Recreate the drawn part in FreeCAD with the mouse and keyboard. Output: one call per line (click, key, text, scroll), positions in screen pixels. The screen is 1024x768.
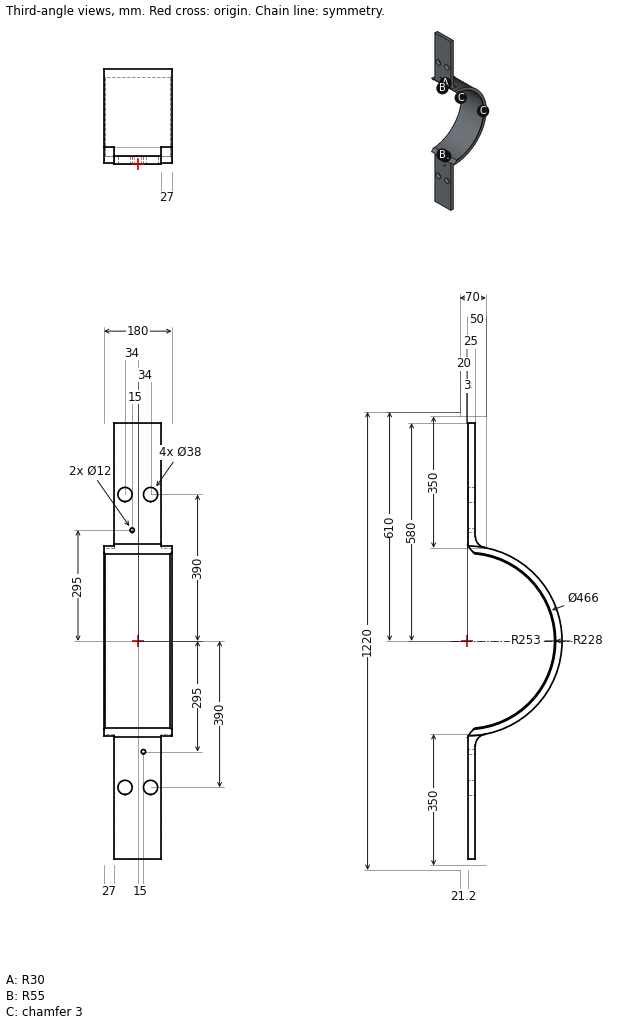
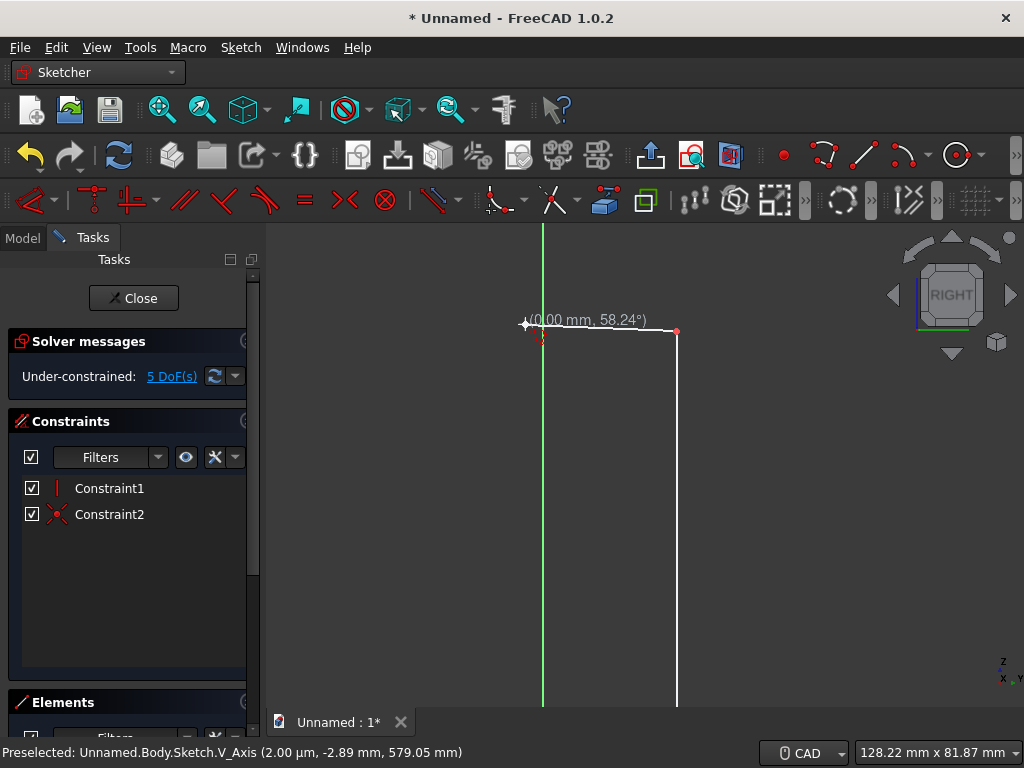
scroll(540, 293, down, 15)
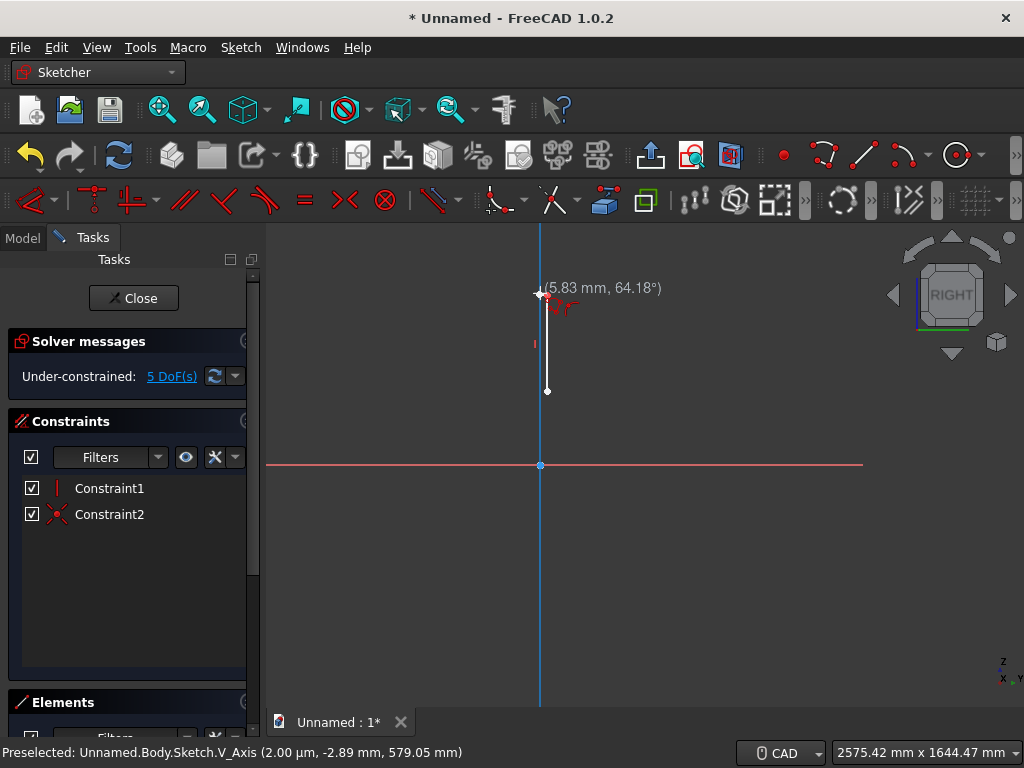
scroll(540, 398, up, 15)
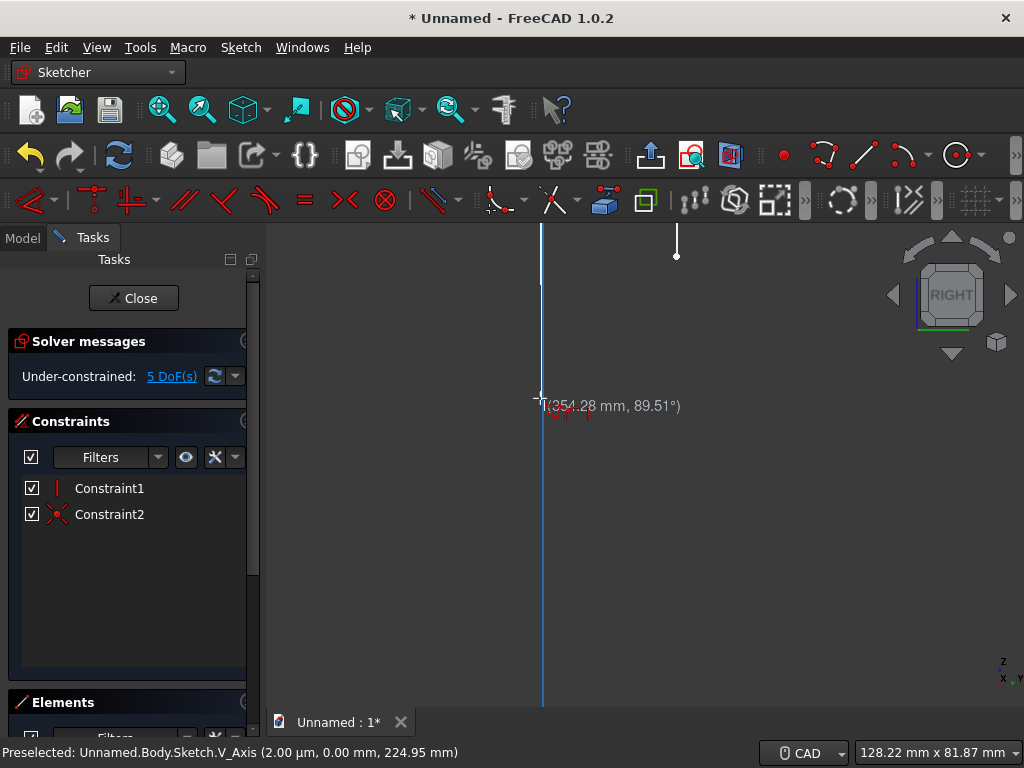
click(525, 393)
right_click(525, 393)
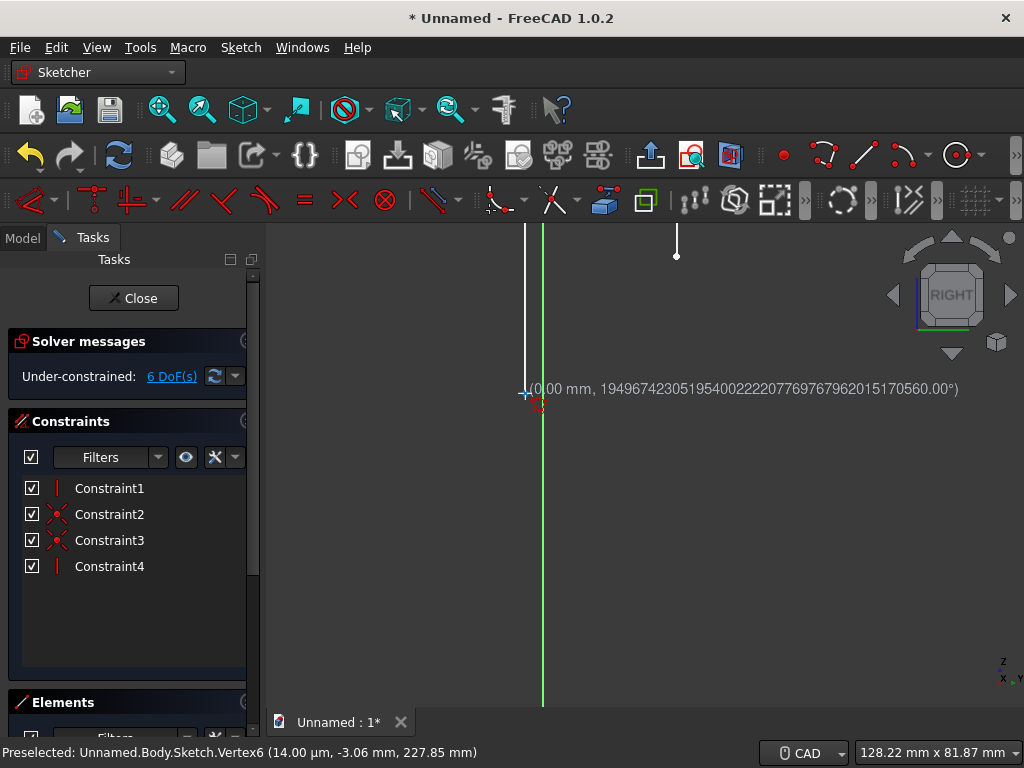
scroll(540, 398, down, 15)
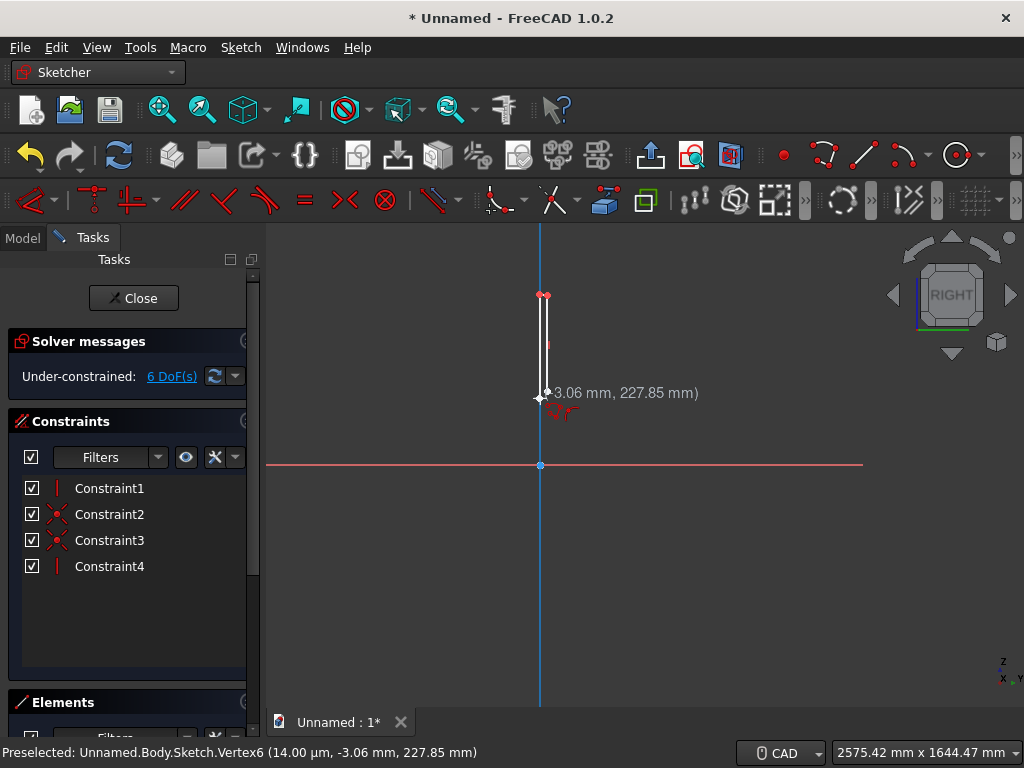
scroll(540, 532, up, 15)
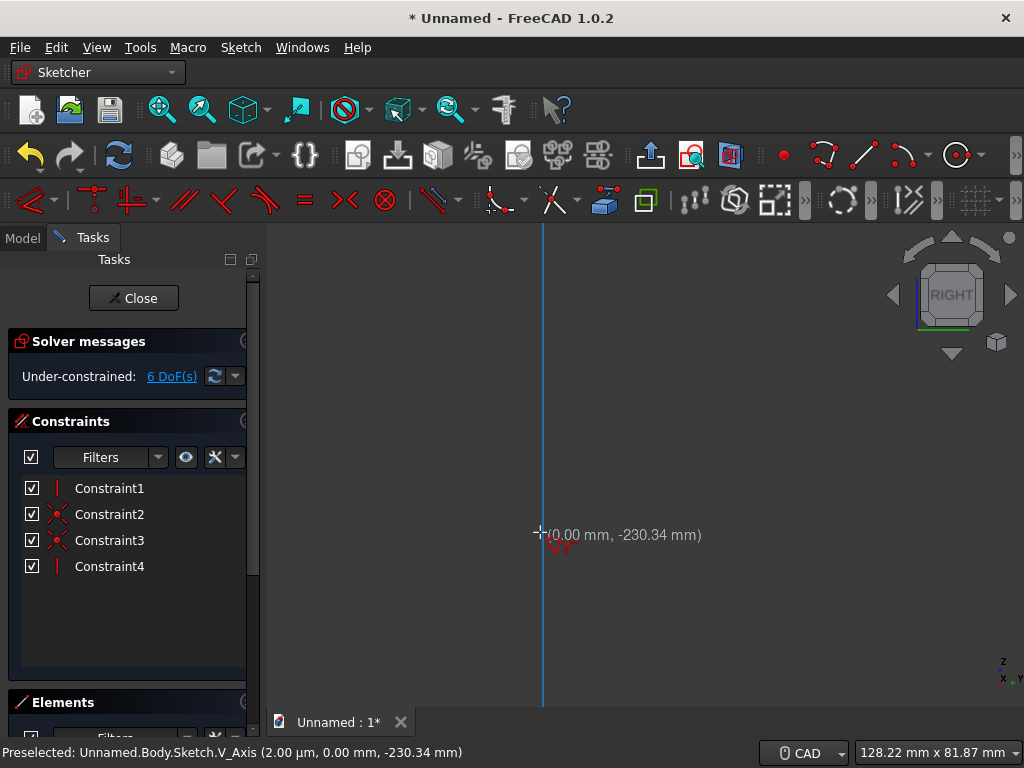
click(525, 526)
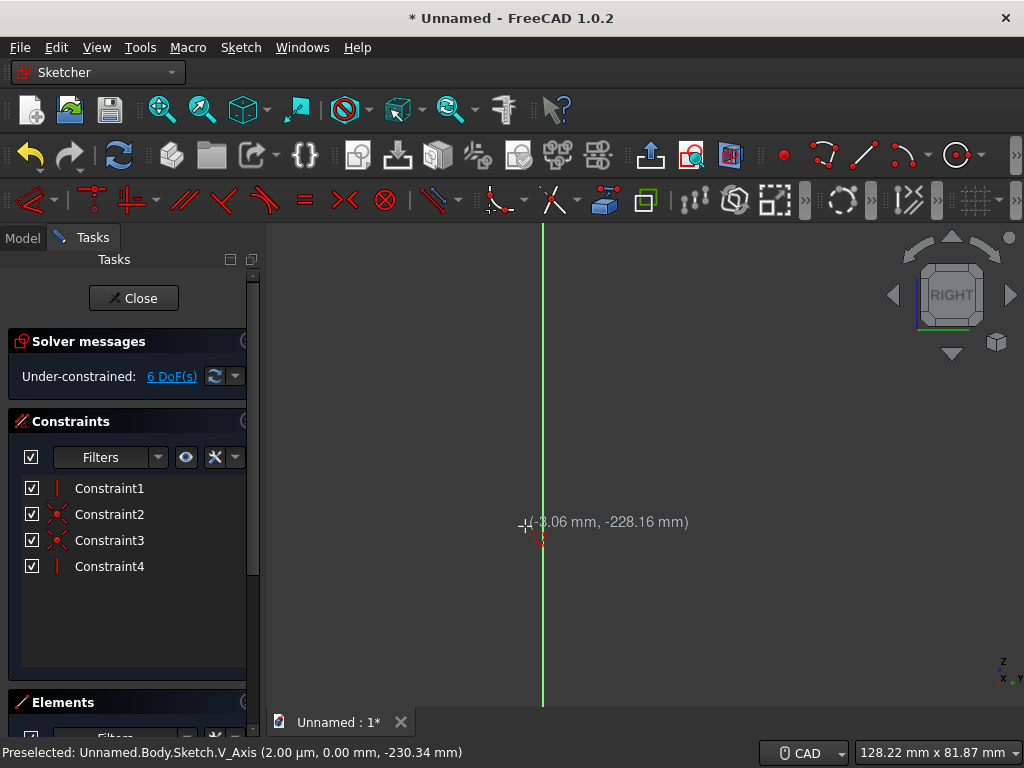
scroll(540, 532, down, 15)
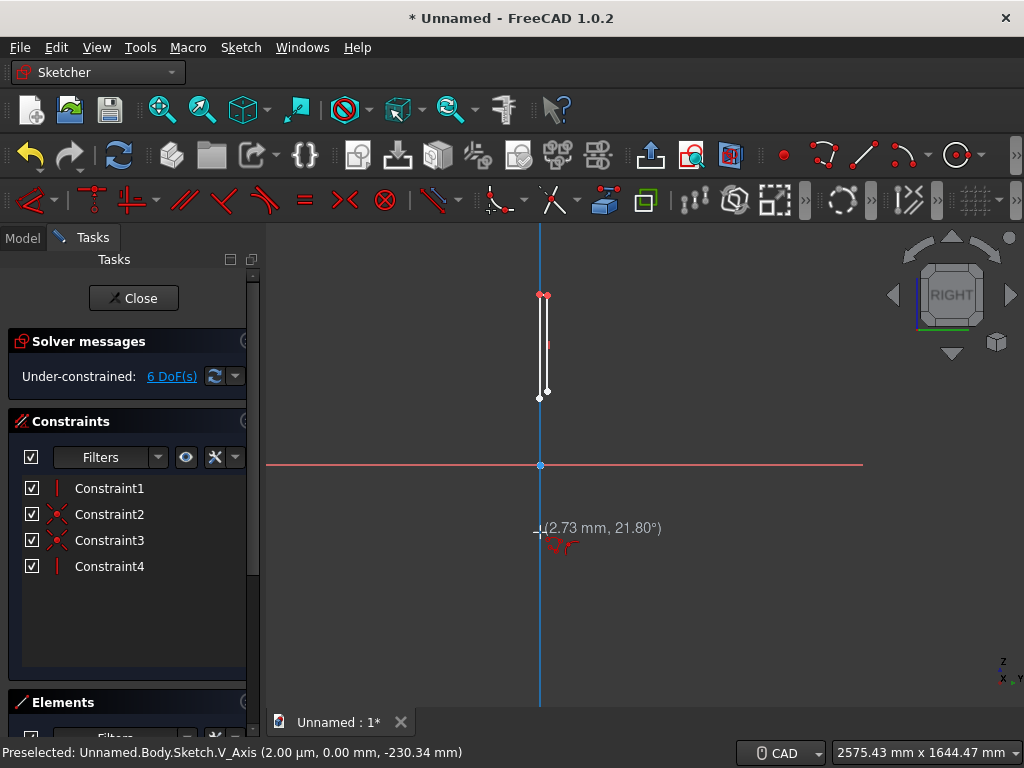
scroll(540, 636, up, 15)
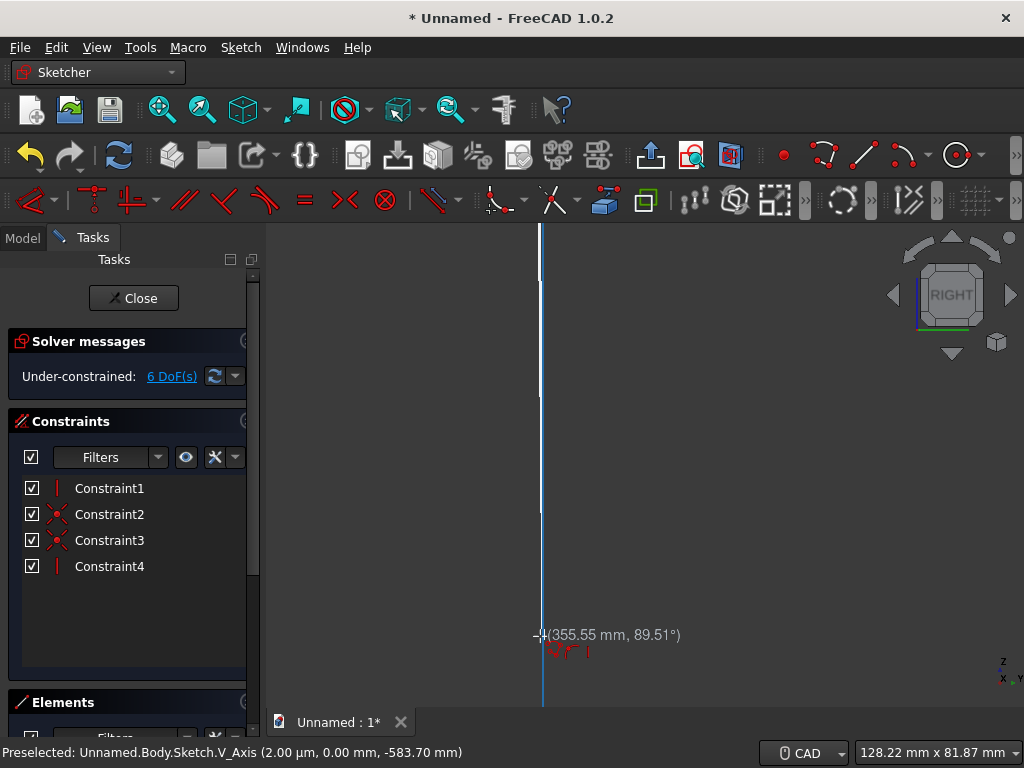
click(525, 618)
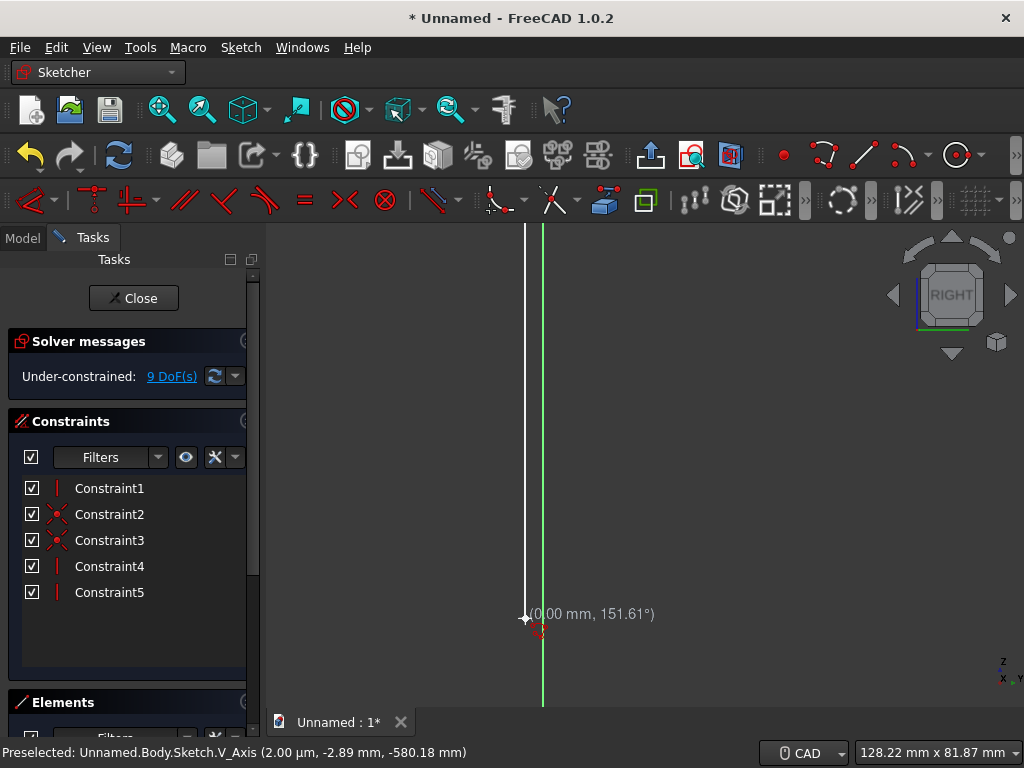
scroll(540, 637, down, 15)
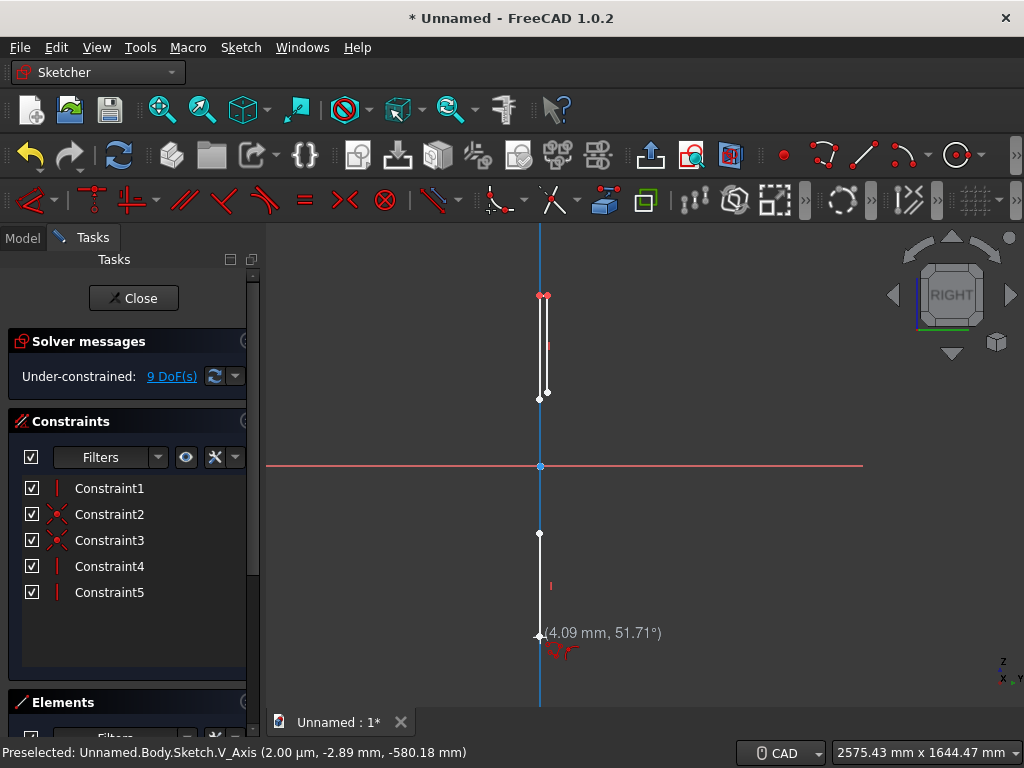
scroll(547, 637, up, 5)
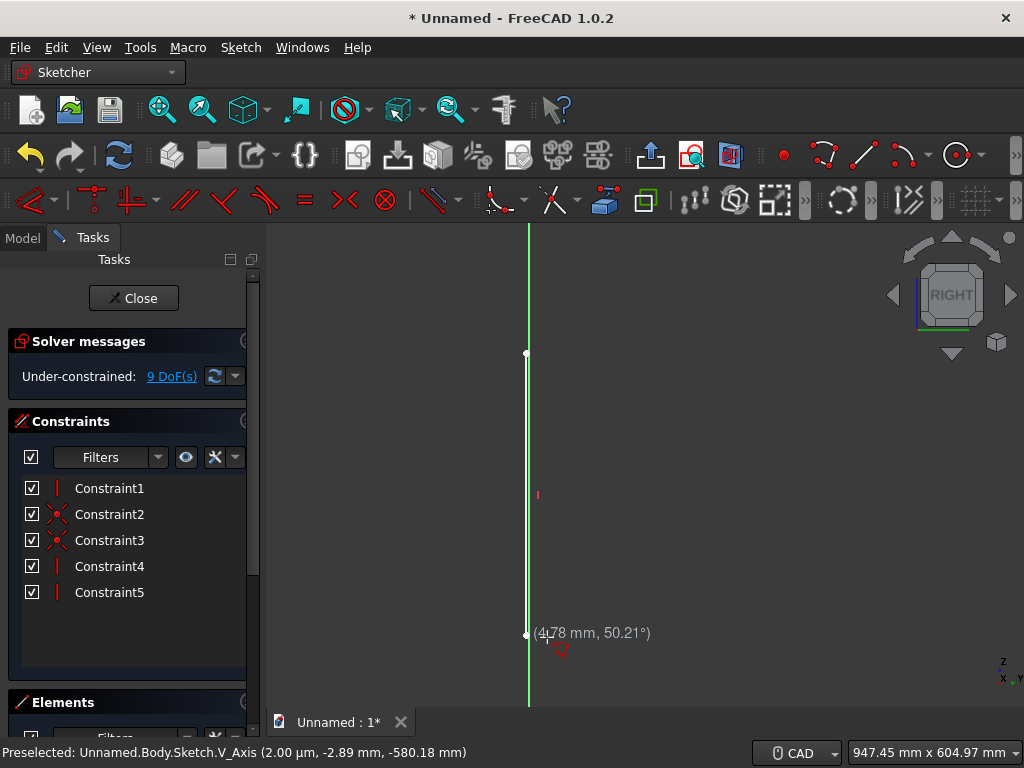
click(546, 635)
click(546, 373)
right_click(546, 373)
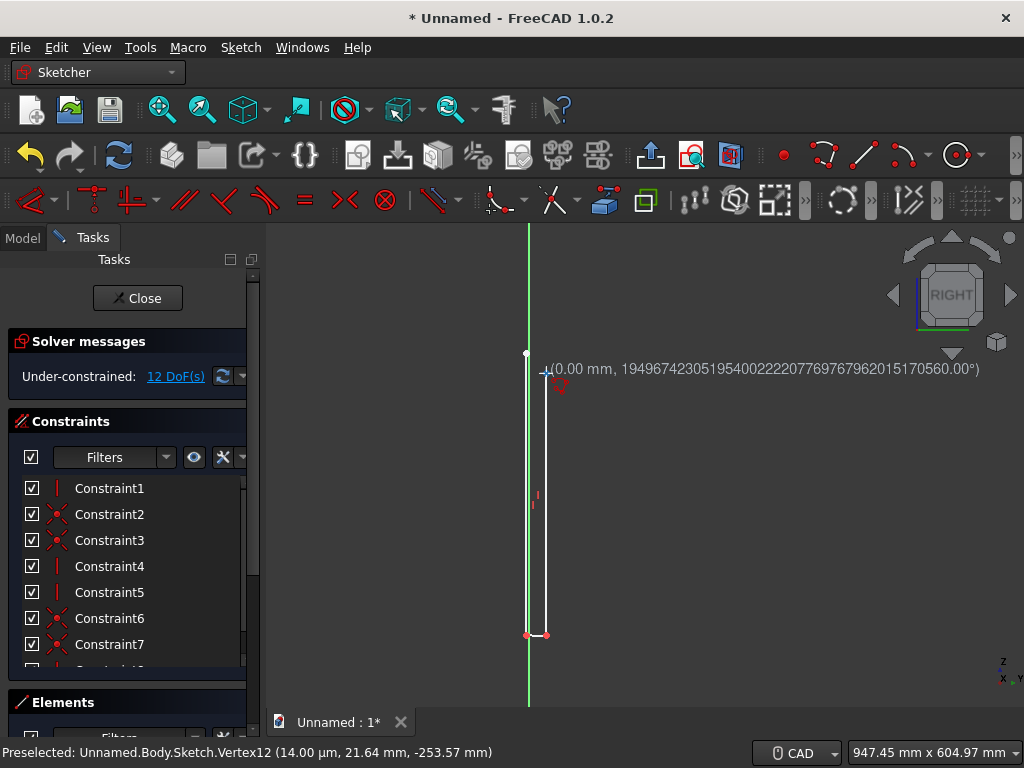
click(930, 156)